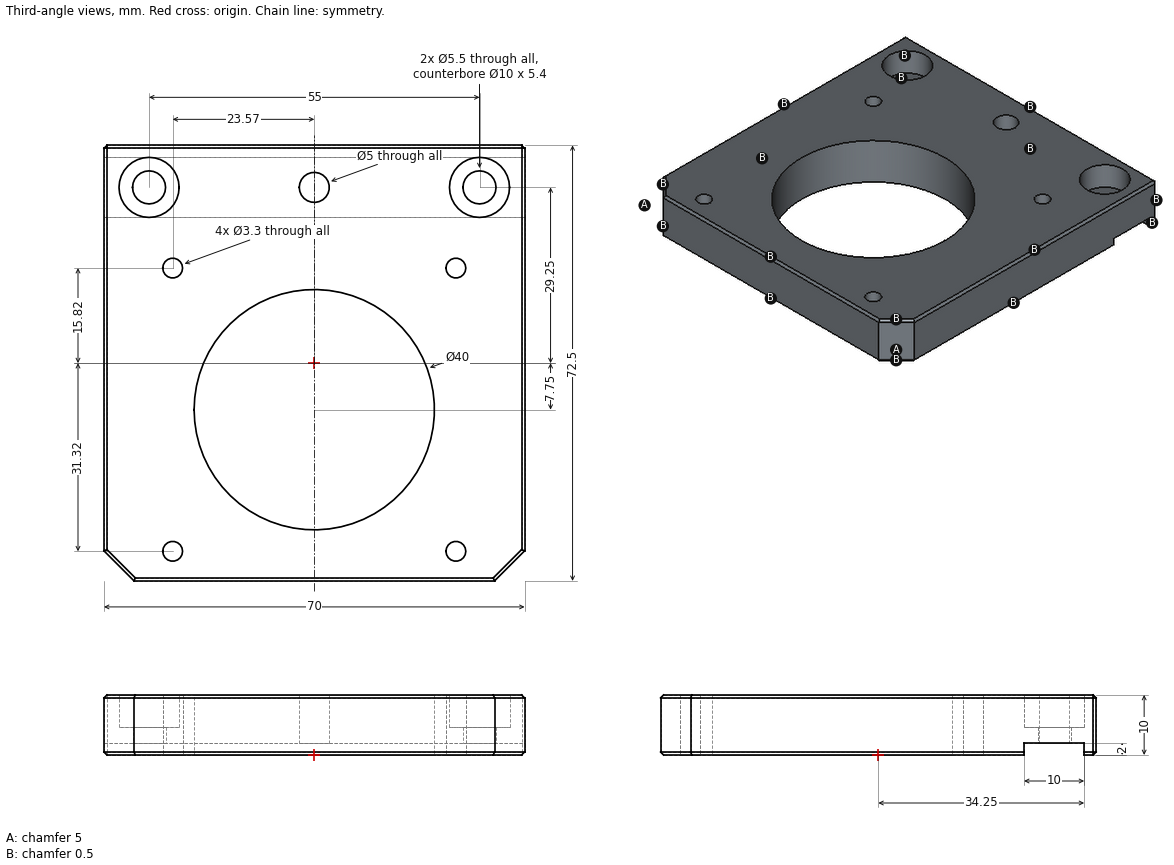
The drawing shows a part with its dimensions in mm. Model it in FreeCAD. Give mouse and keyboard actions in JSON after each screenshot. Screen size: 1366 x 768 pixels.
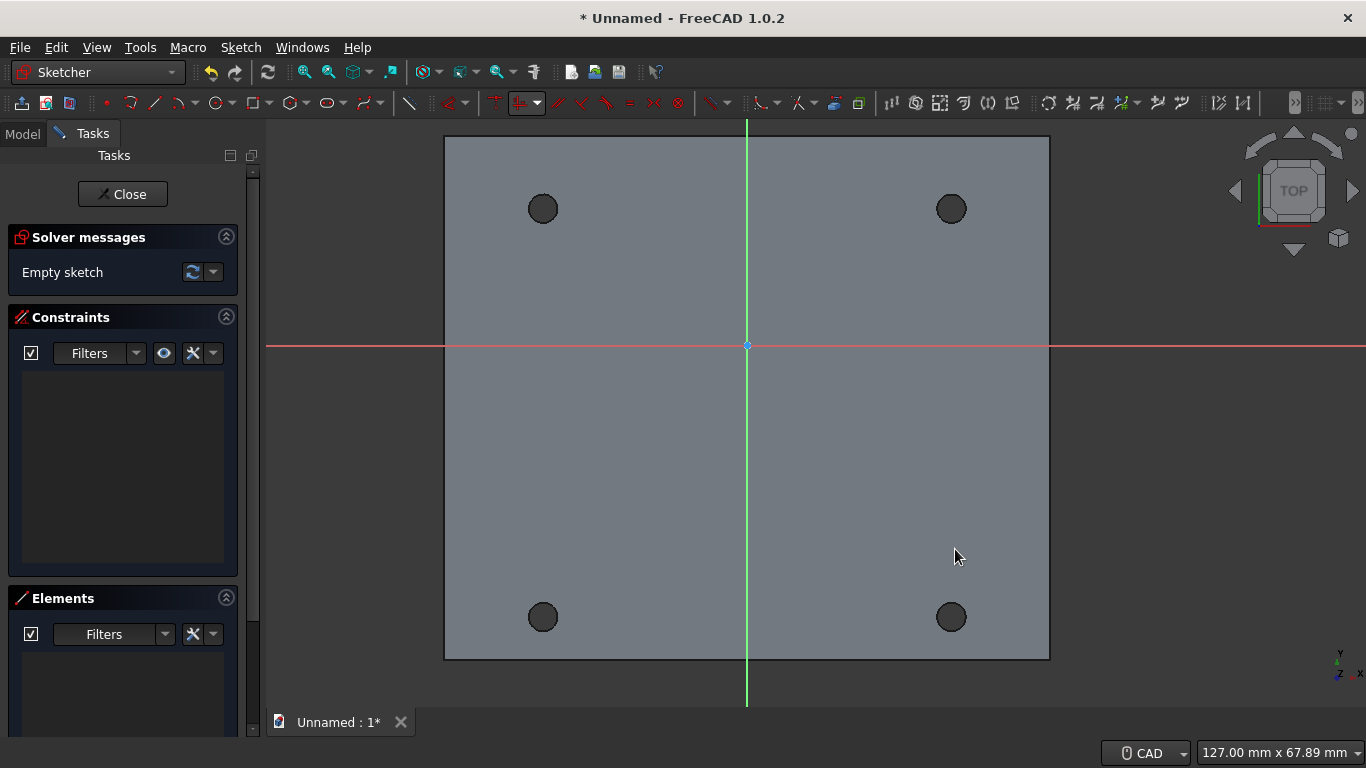
{"action": "left_click", "coordinate": [216, 104]}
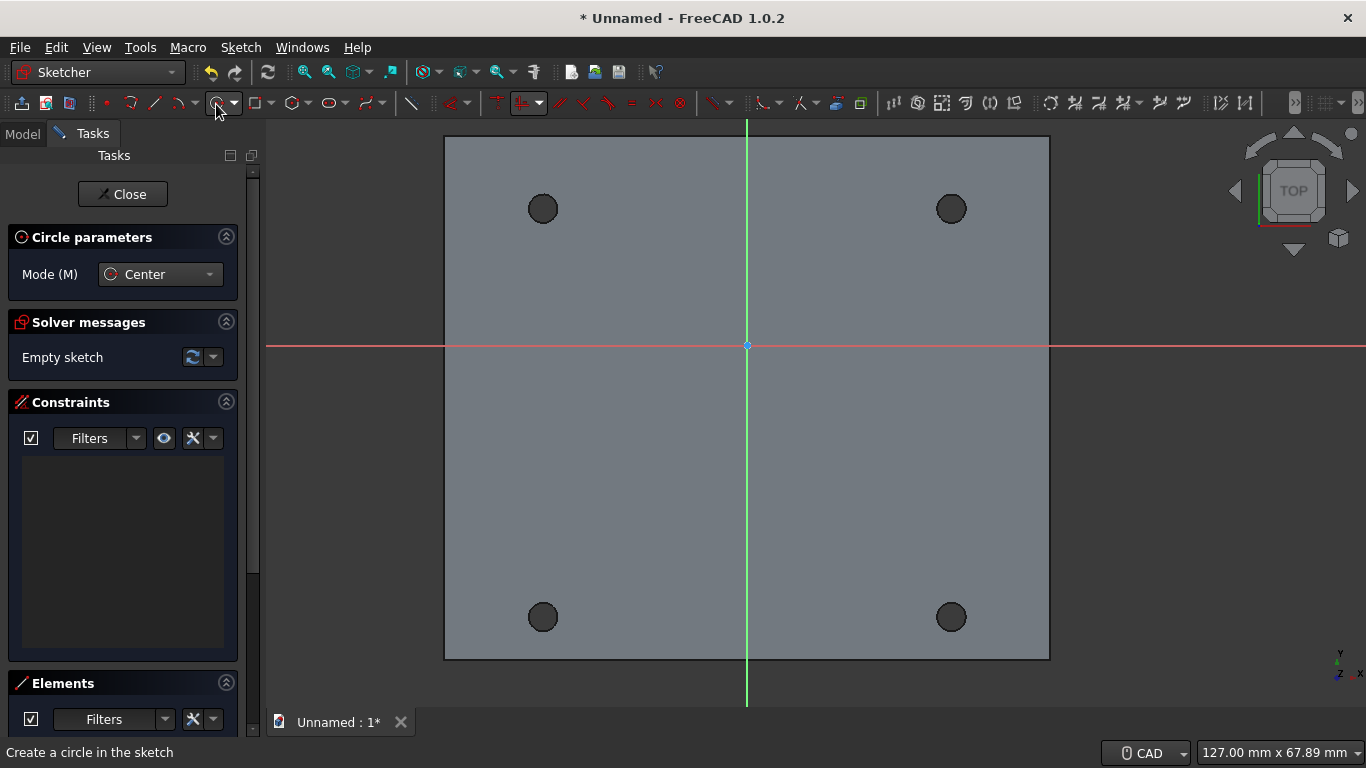
{"action": "left_click", "coordinate": [747, 413]}
{"action": "mouse_move", "coordinate": [870, 290]}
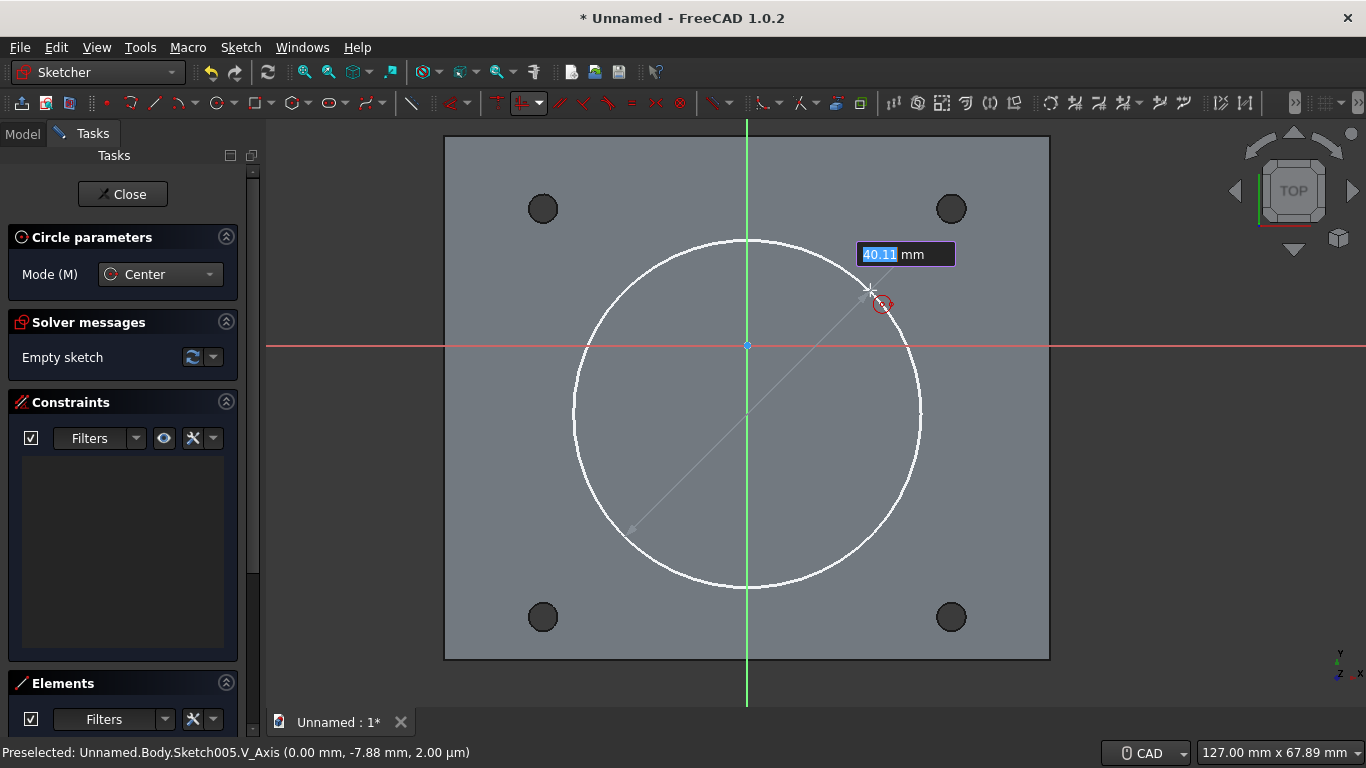
{"action": "type", "text": "40"}
{"action": "key", "text": "Return"}
{"action": "key", "text": "Escape"}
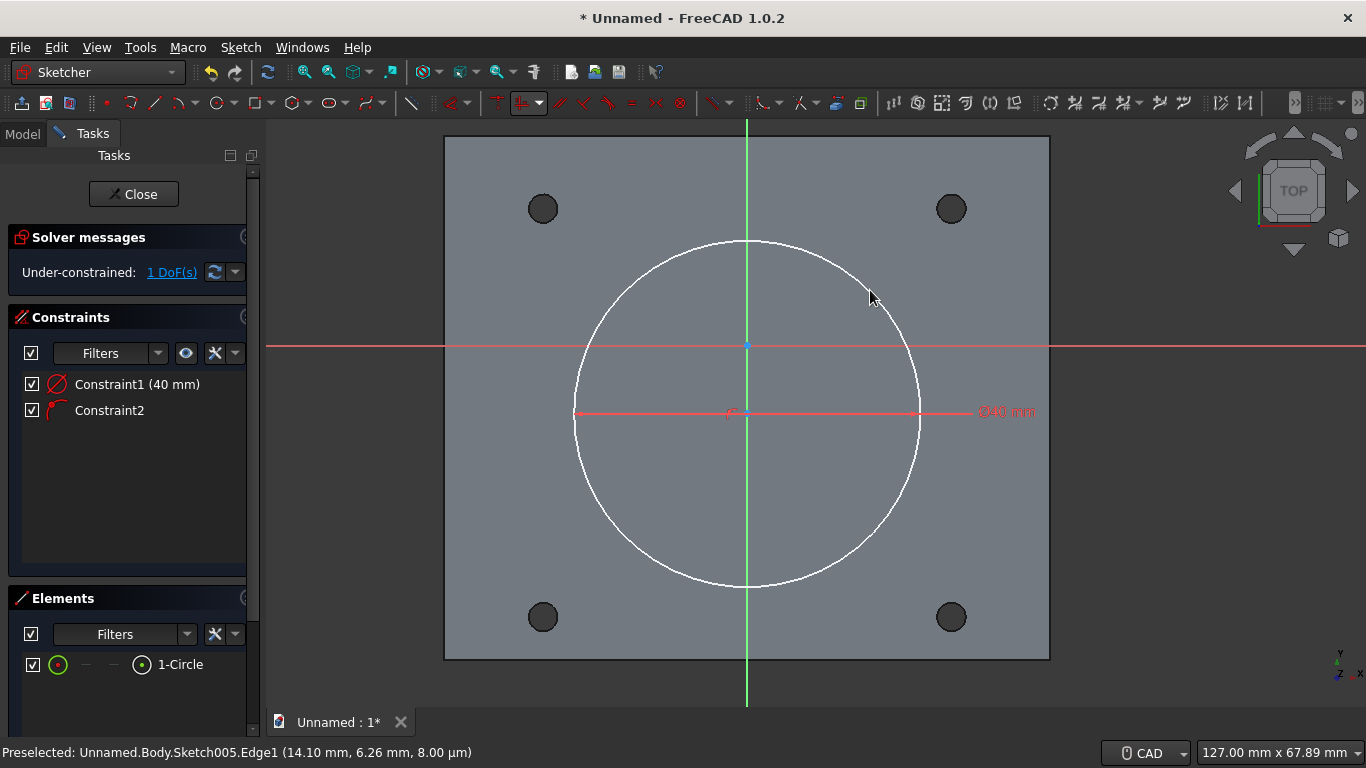
{"action": "left_click", "coordinate": [450, 104]}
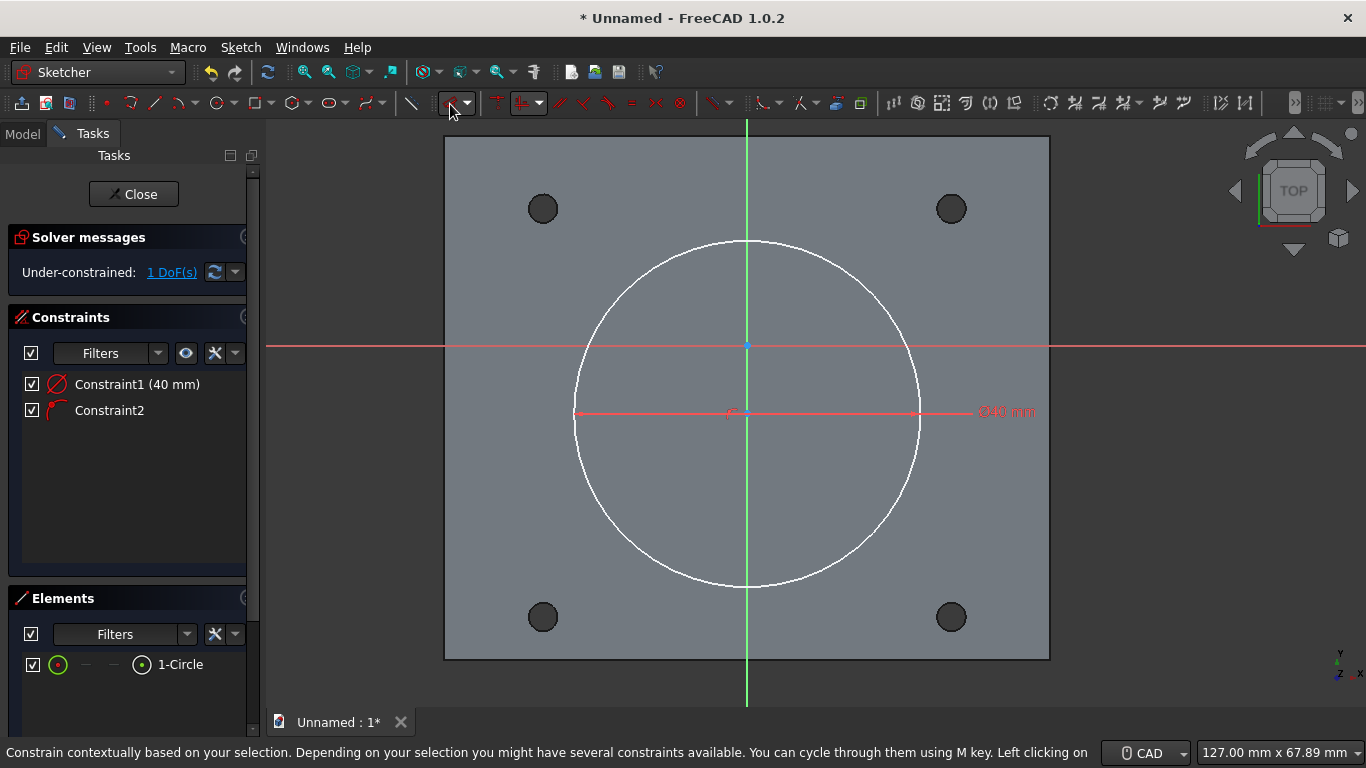
{"action": "left_click", "coordinate": [747, 414]}
{"action": "left_click", "coordinate": [781, 380]}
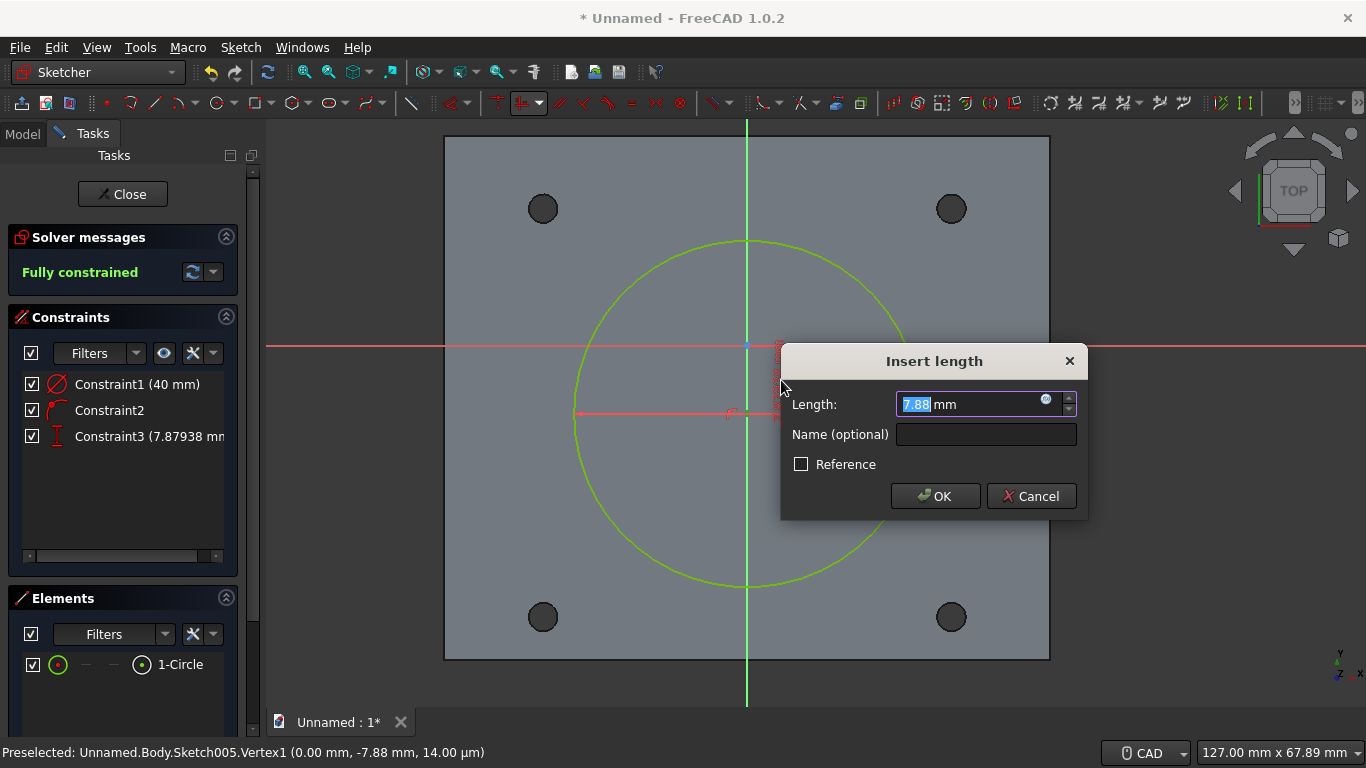
{"action": "type", "text": "7.75"}
{"action": "key", "text": "Return"}
{"action": "key", "text": "Escape"}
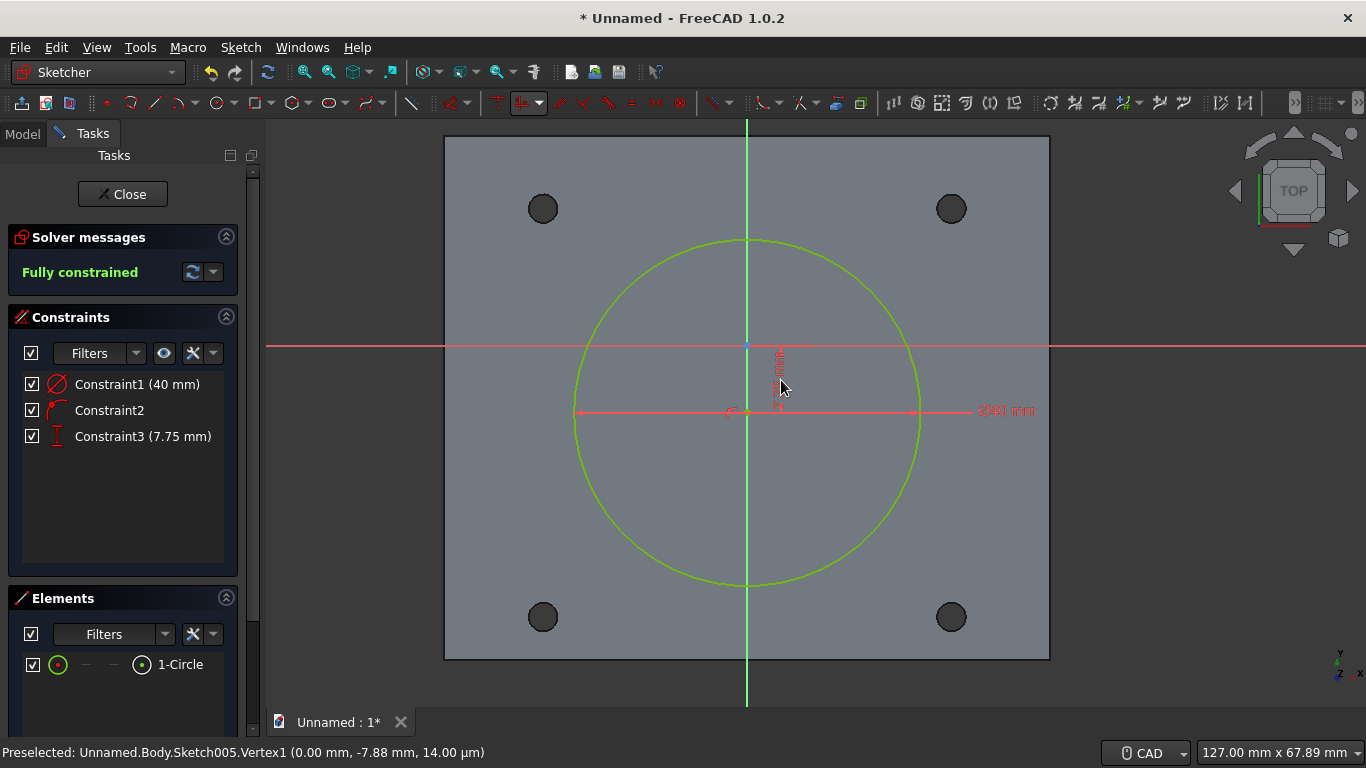
{"action": "left_click", "coordinate": [123, 194]}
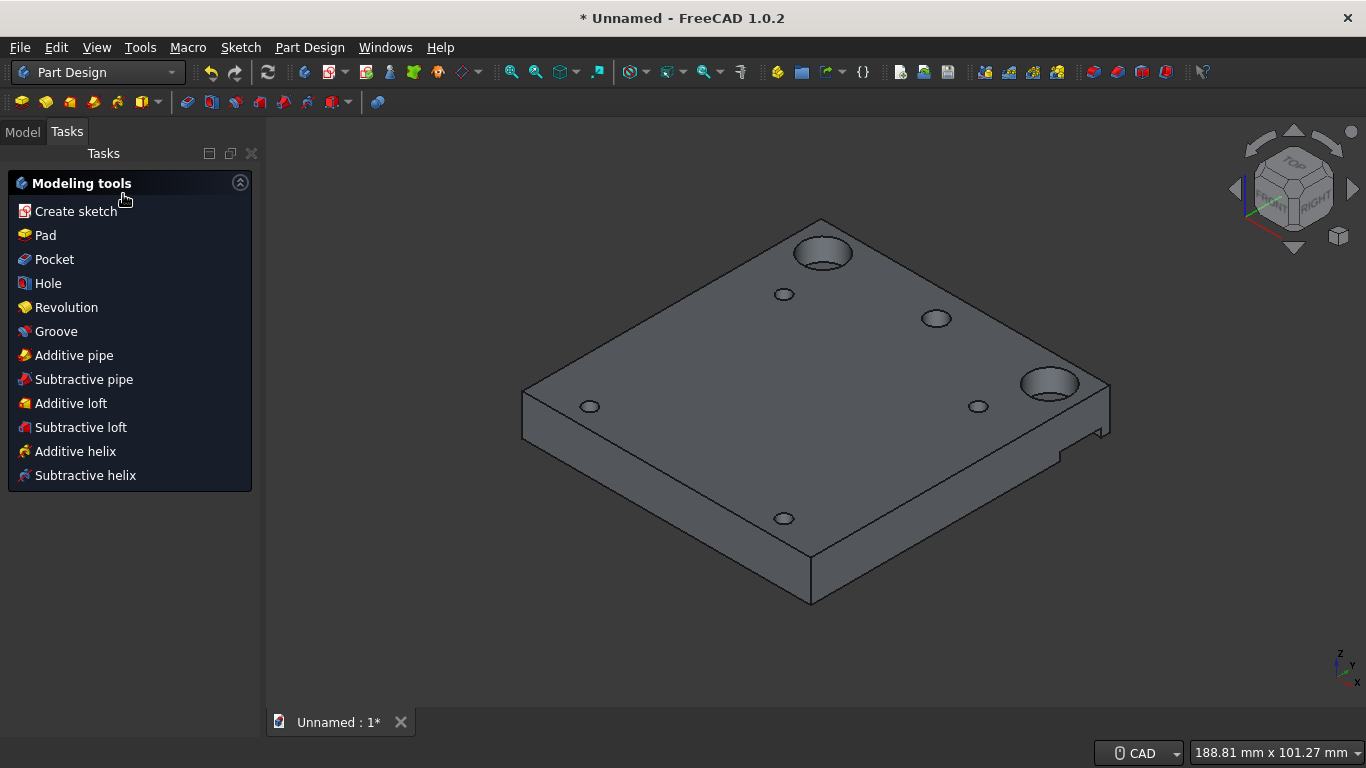
{"action": "left_click", "coordinate": [188, 102]}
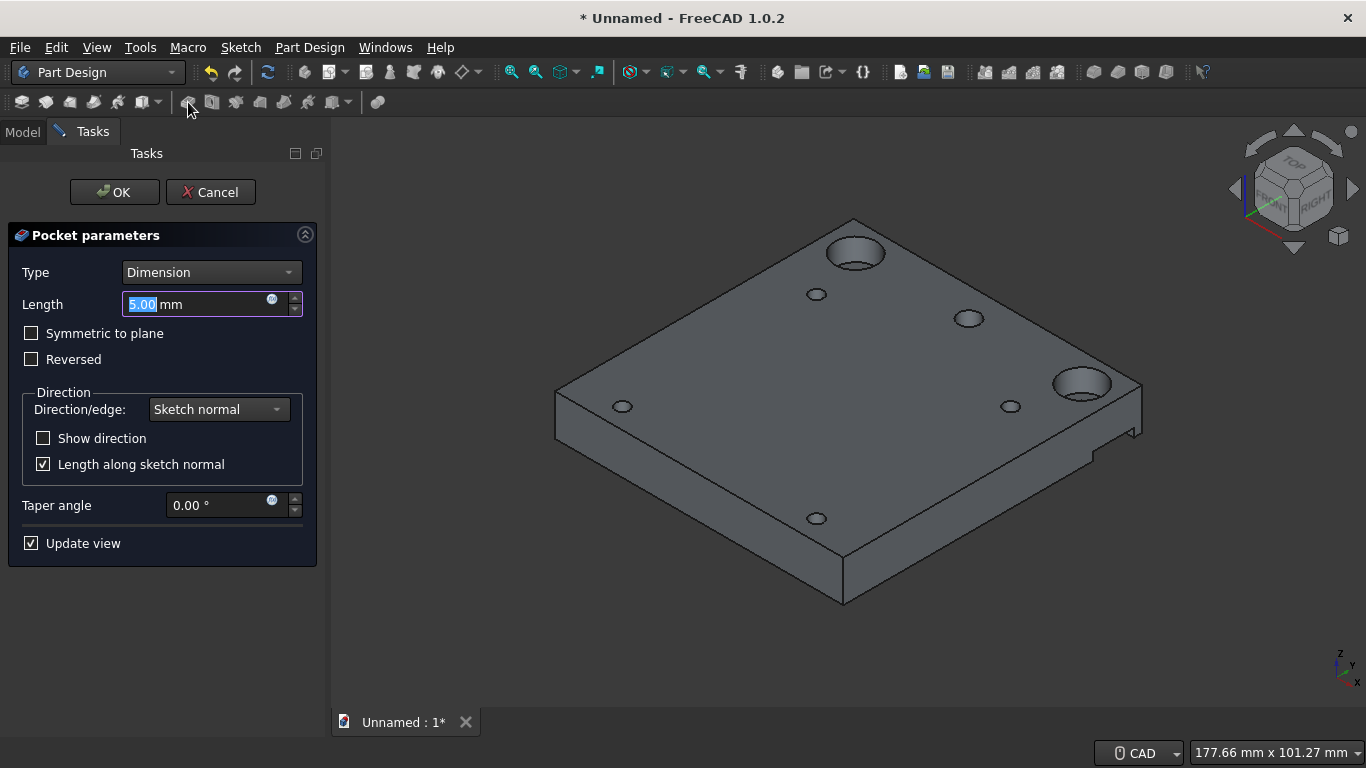
{"action": "left_click", "coordinate": [212, 272]}